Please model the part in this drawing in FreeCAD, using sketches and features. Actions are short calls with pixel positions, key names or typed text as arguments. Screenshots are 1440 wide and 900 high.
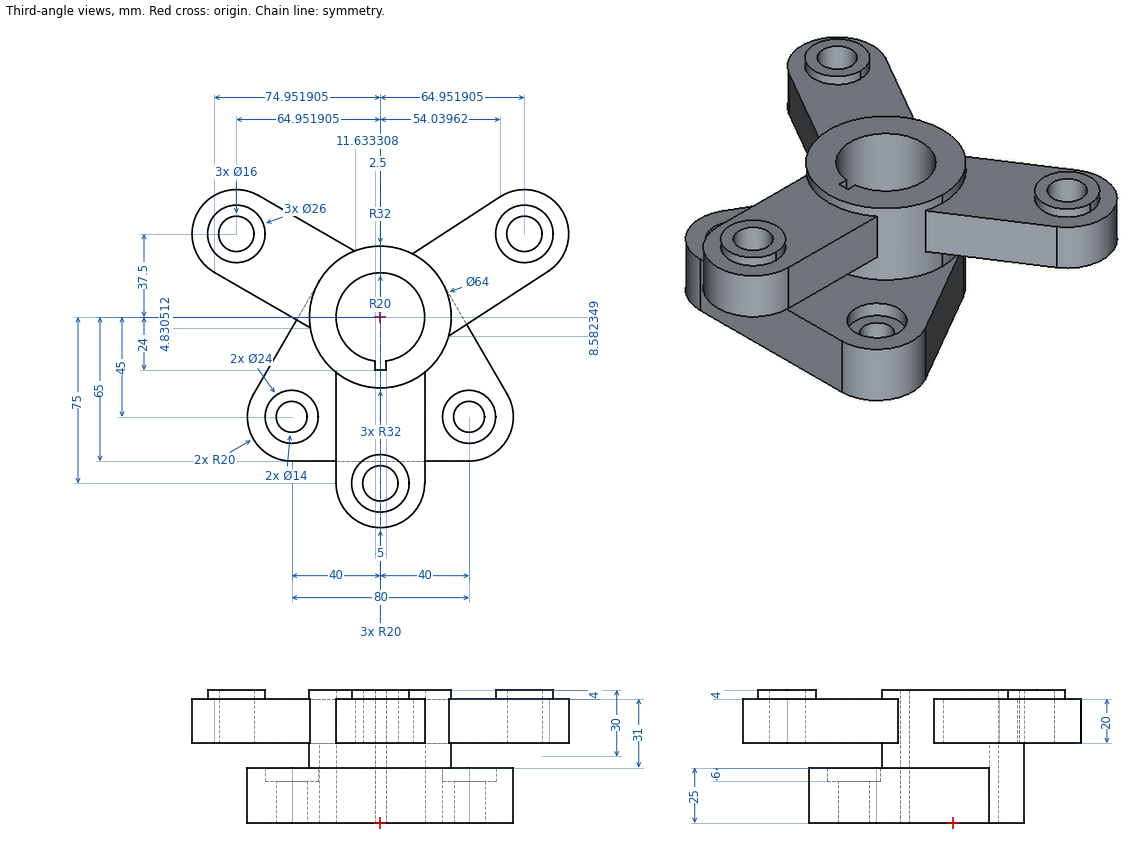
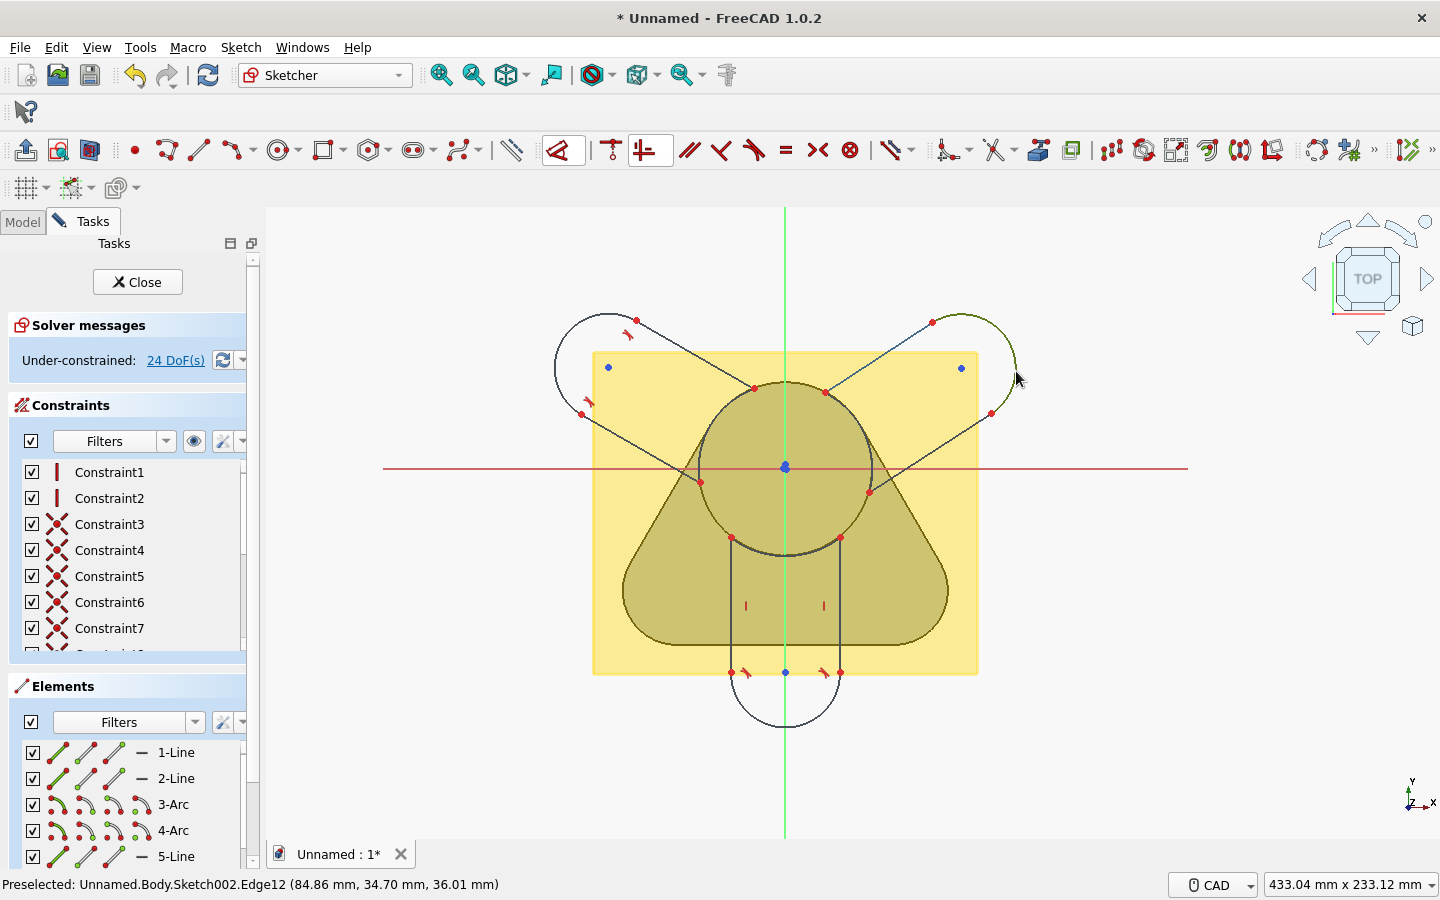
key(t)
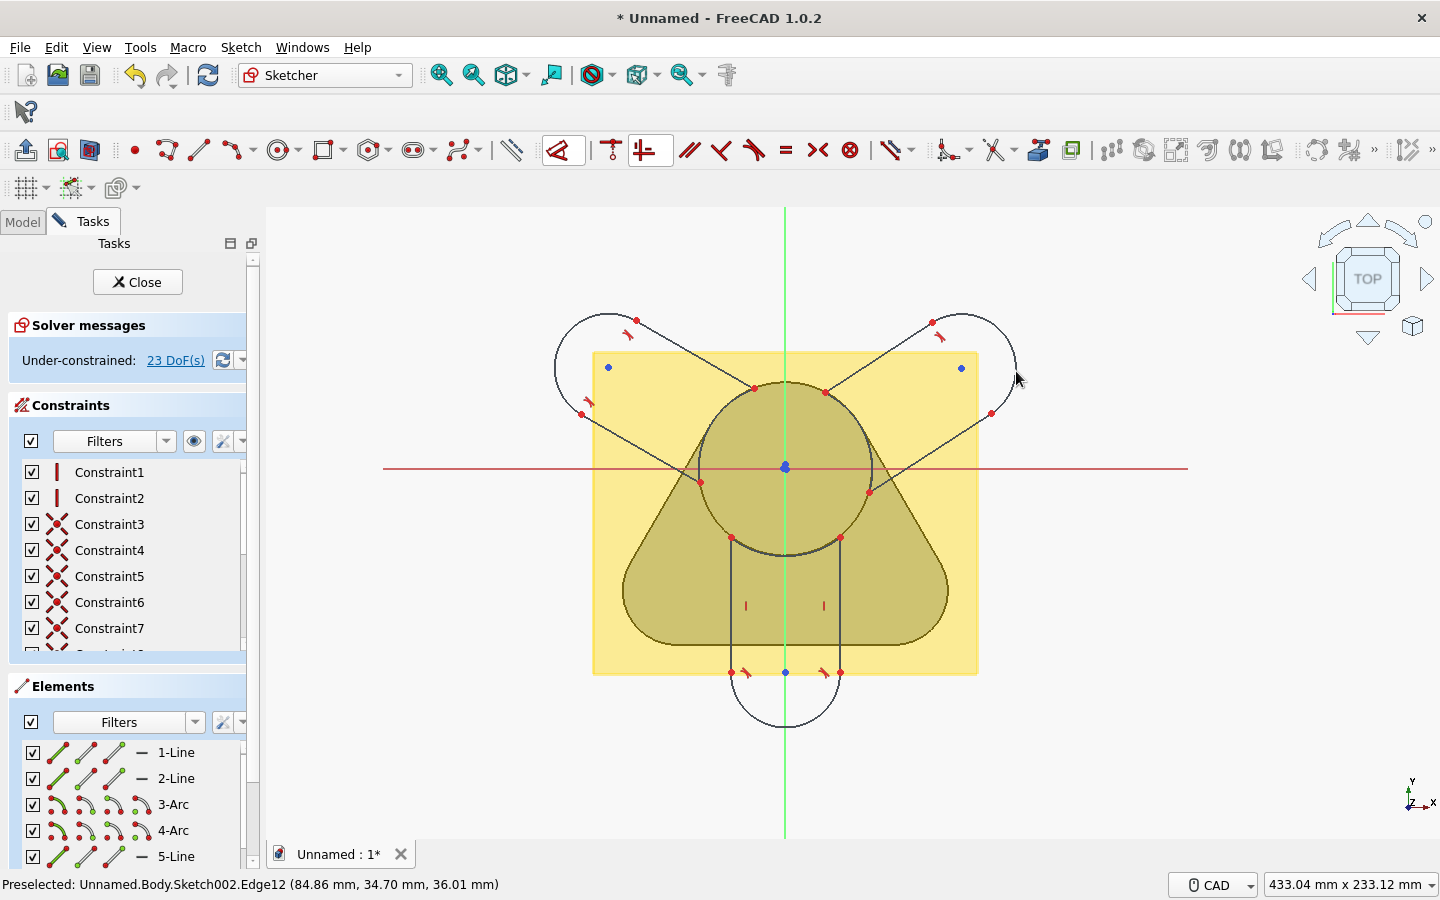
click(906, 469)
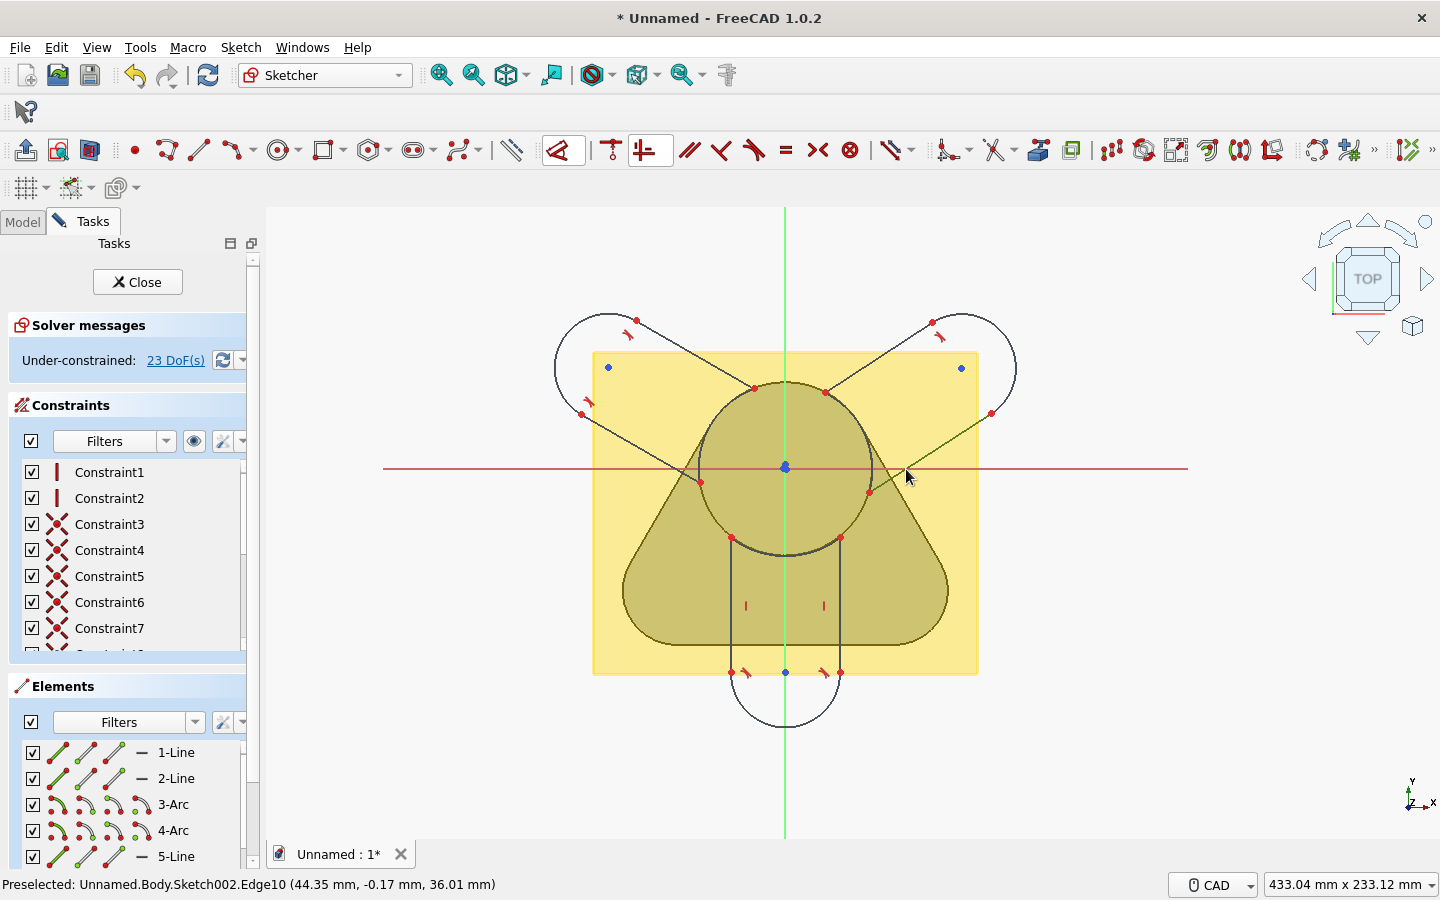
click(1016, 371)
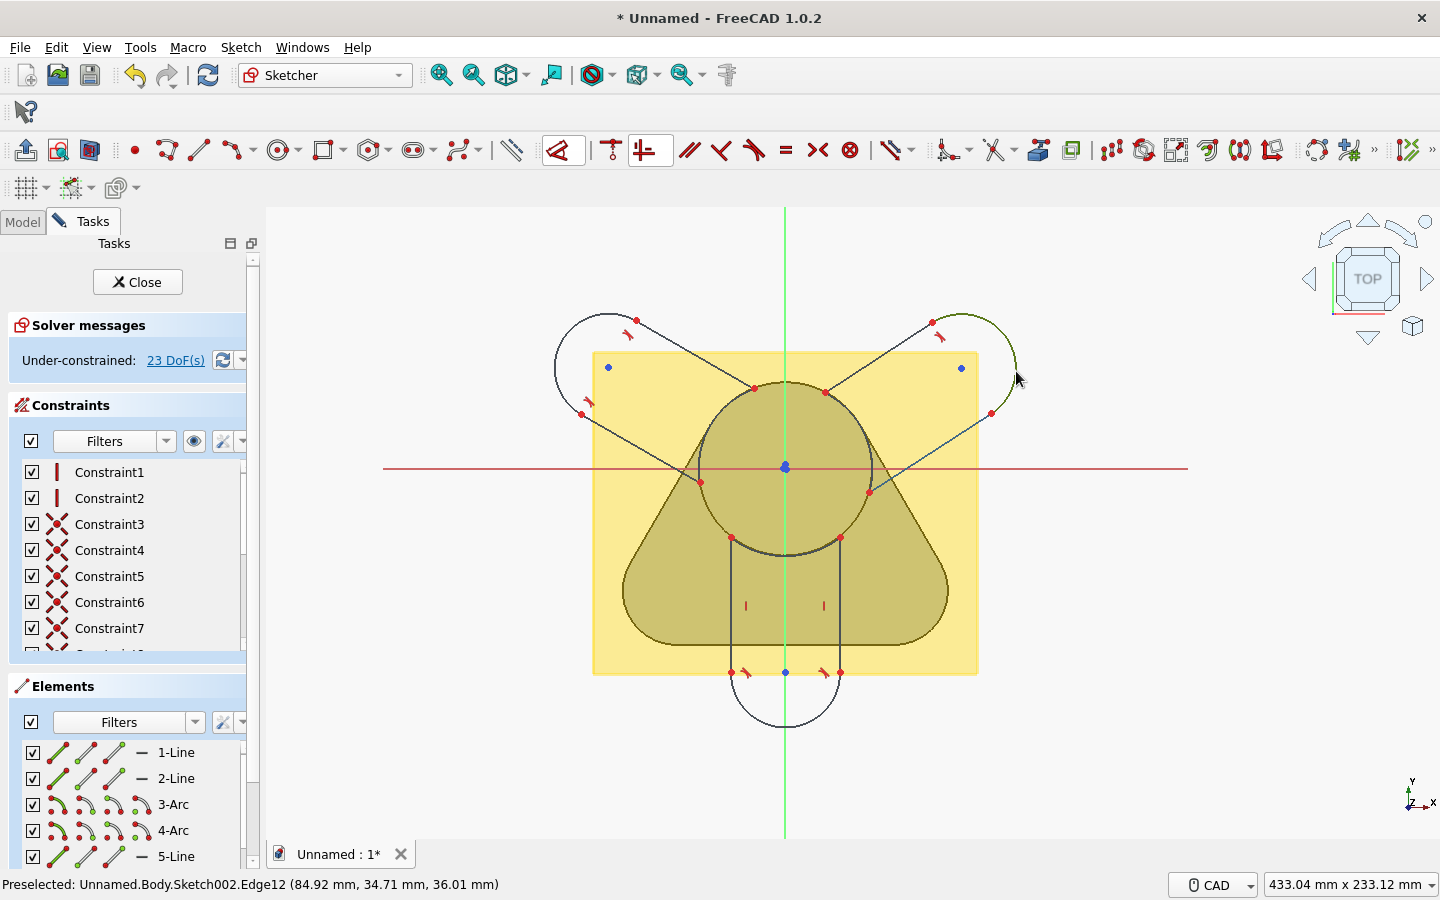
click(754, 150)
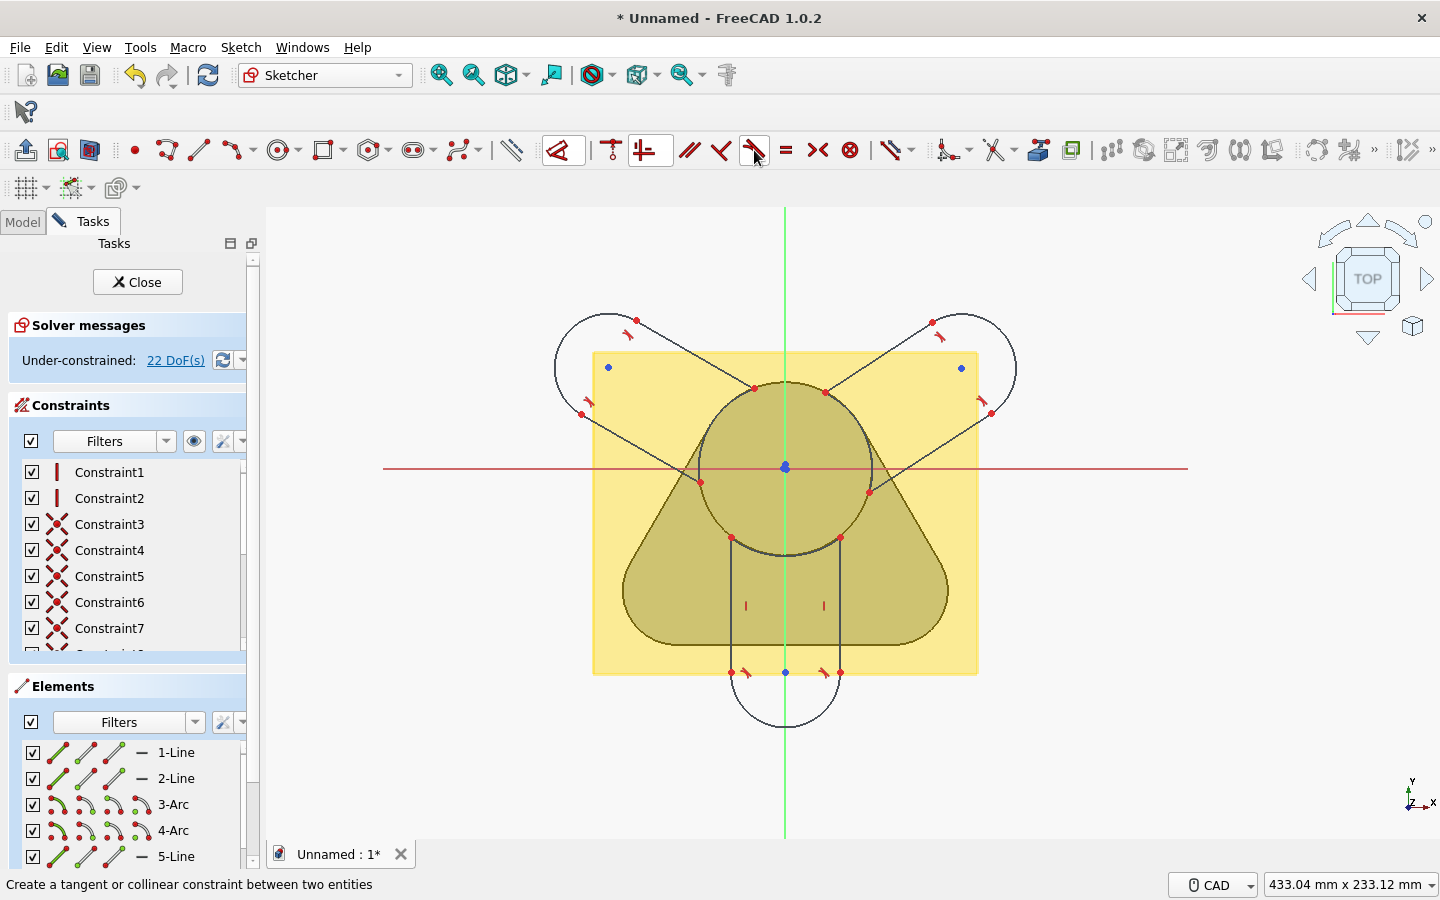
click(762, 553)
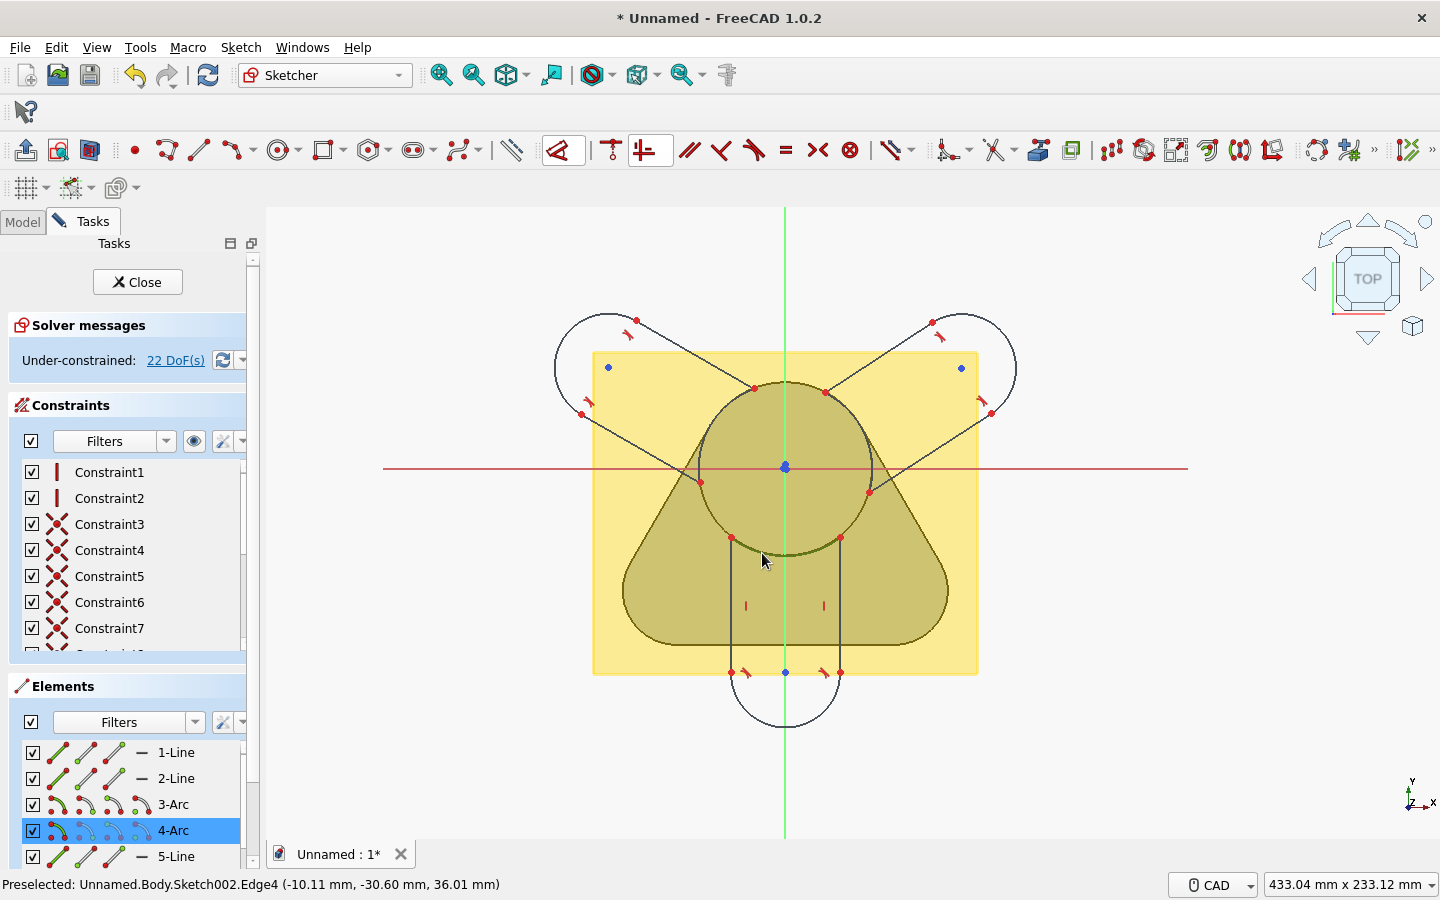
click(724, 408)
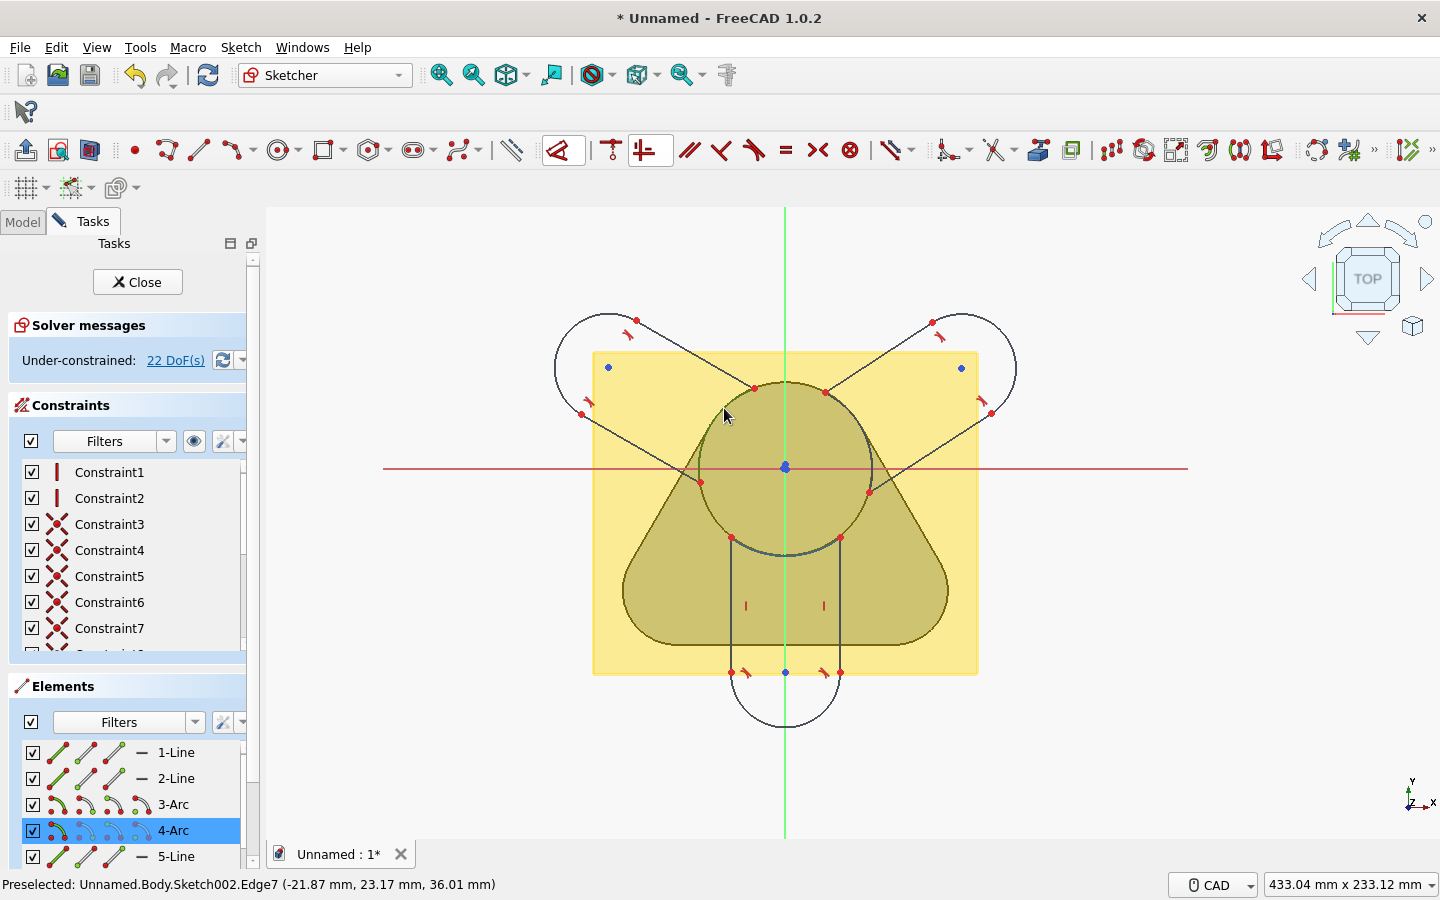
click(612, 150)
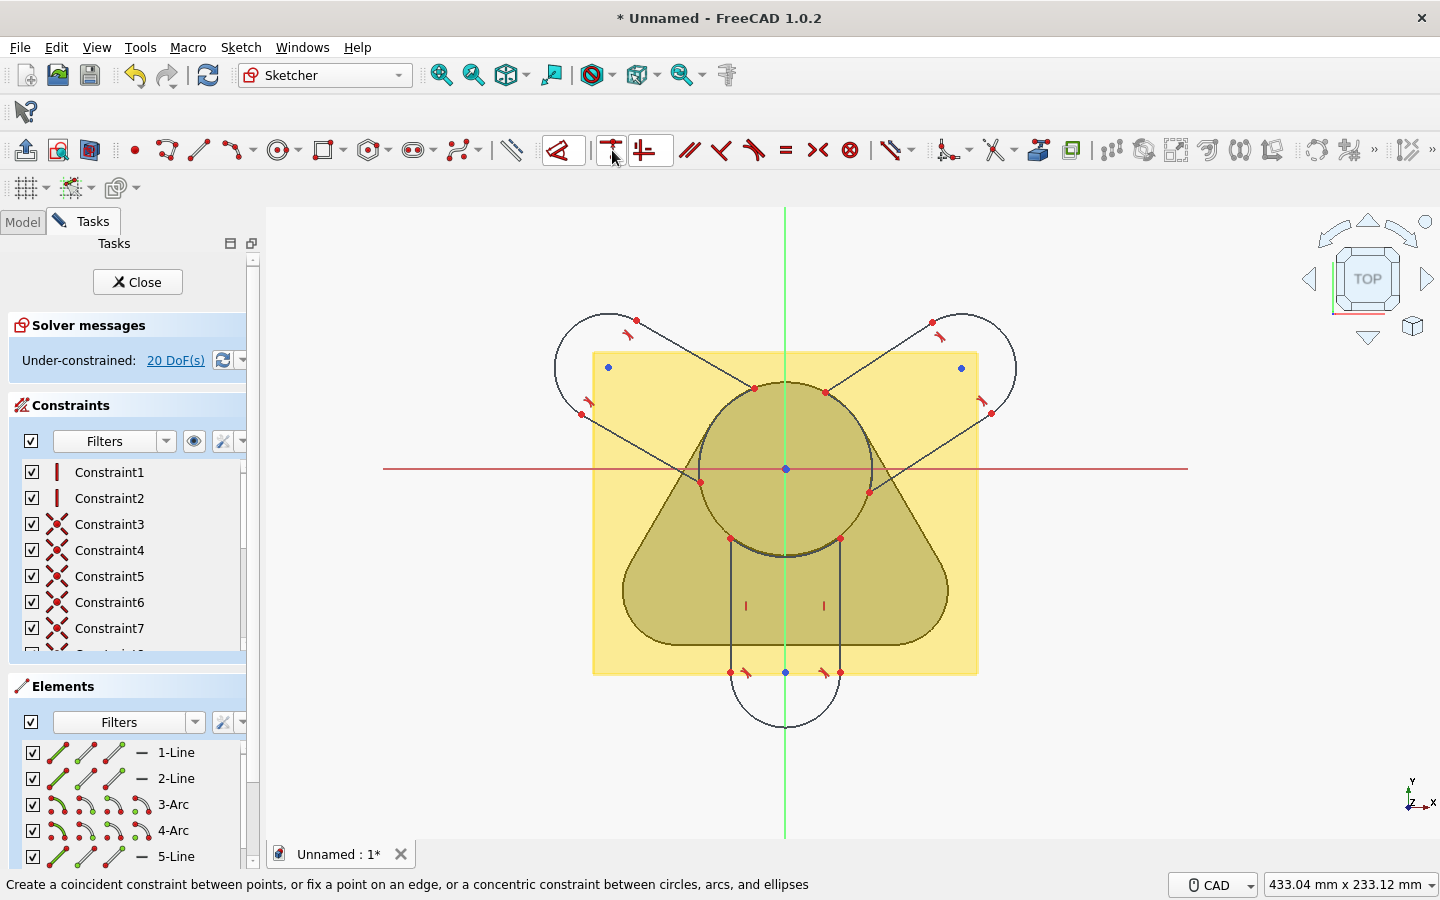
click(762, 554)